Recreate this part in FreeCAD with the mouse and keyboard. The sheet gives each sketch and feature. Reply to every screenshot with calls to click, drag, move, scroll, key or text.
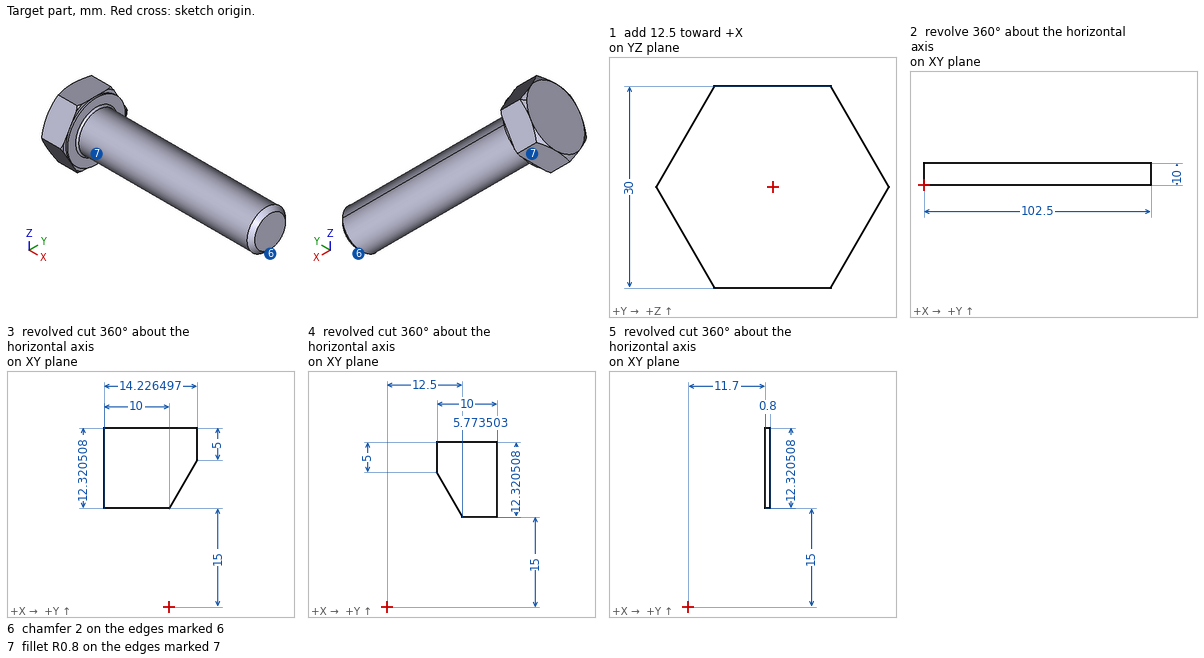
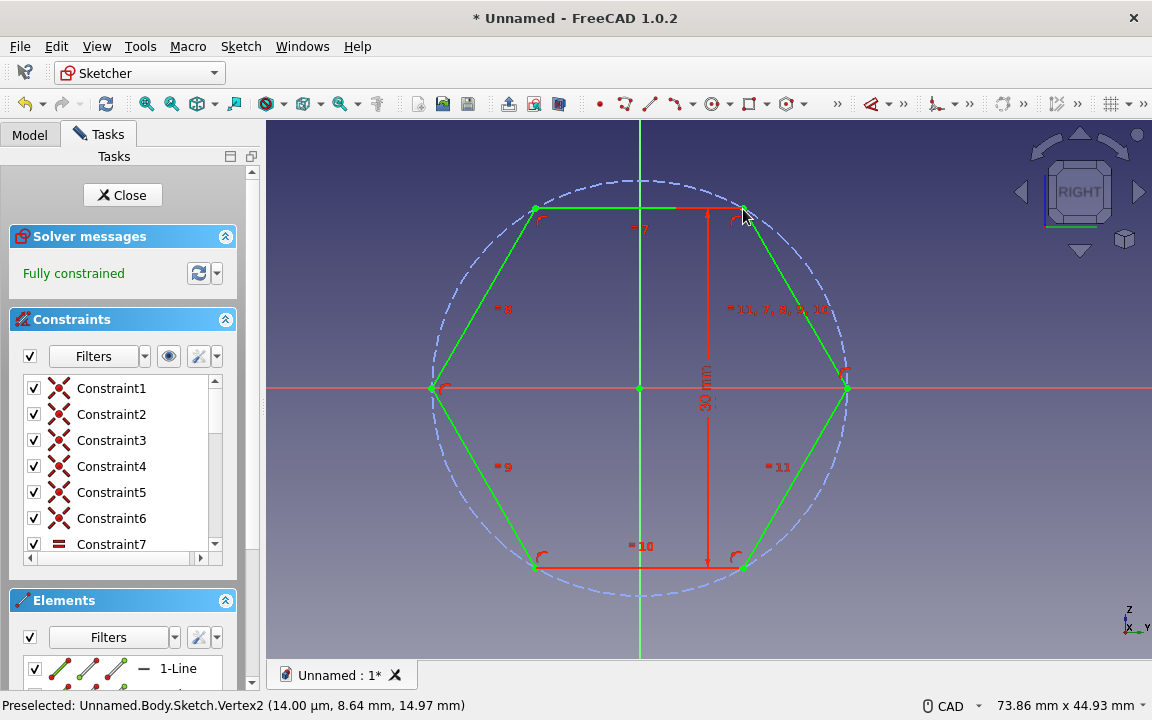
click(123, 195)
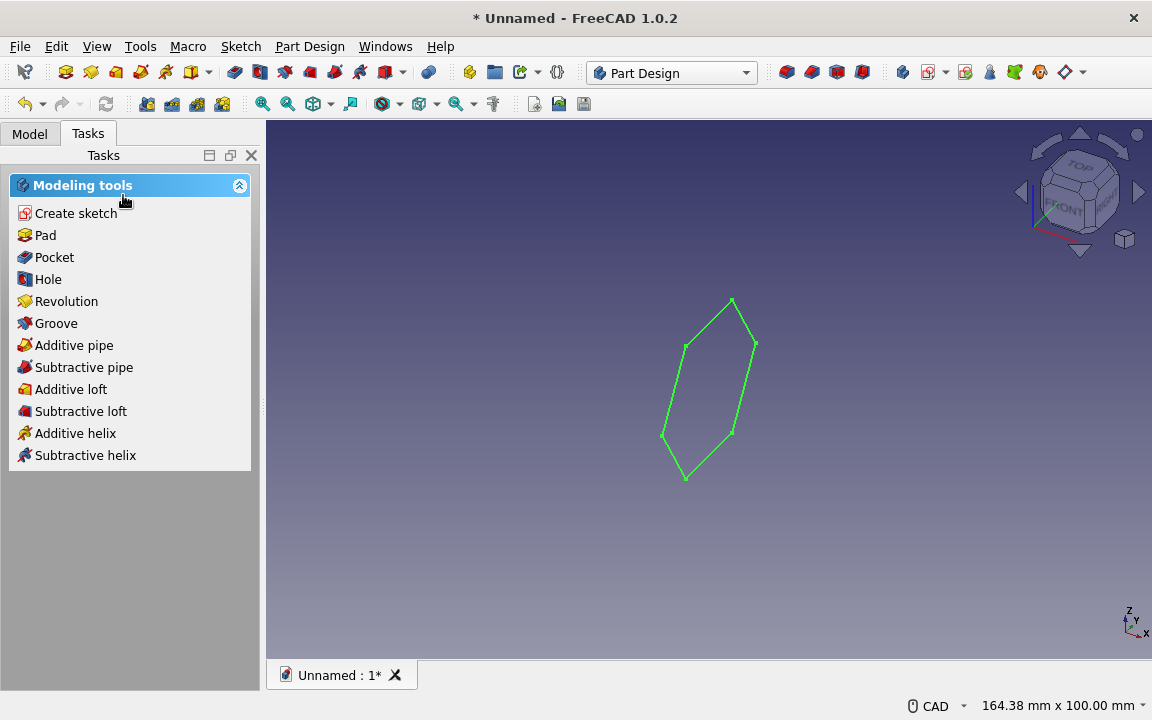
click(66, 72)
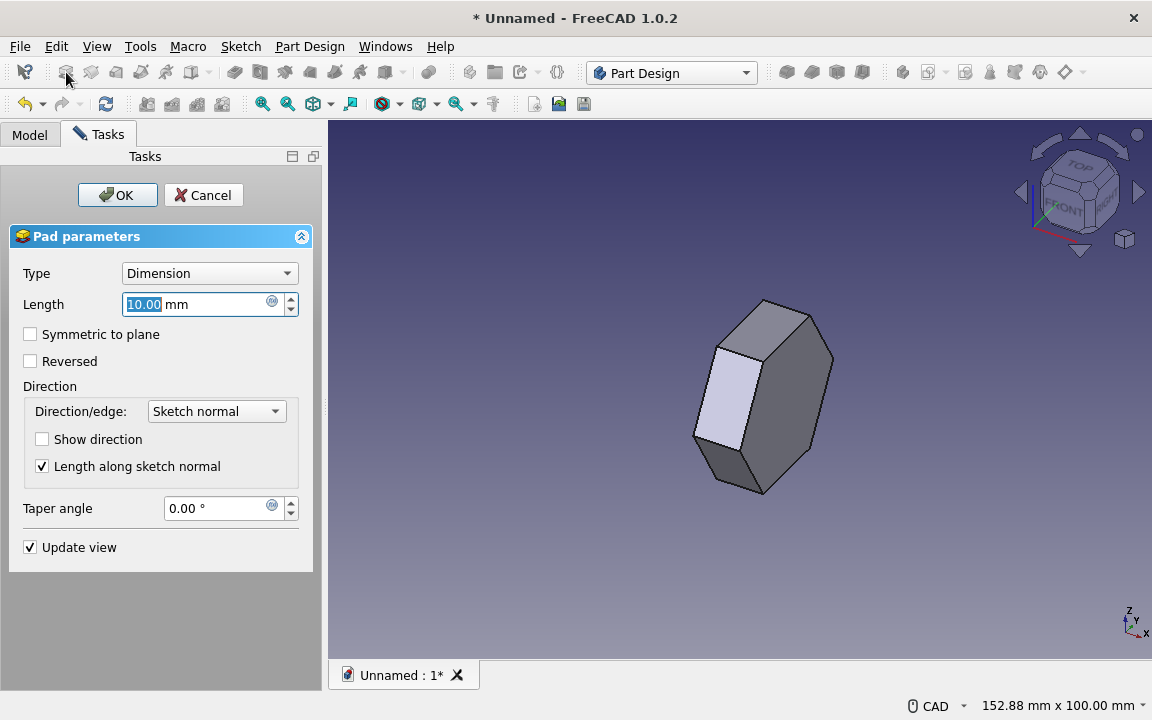
text(12.5)
key(Tab)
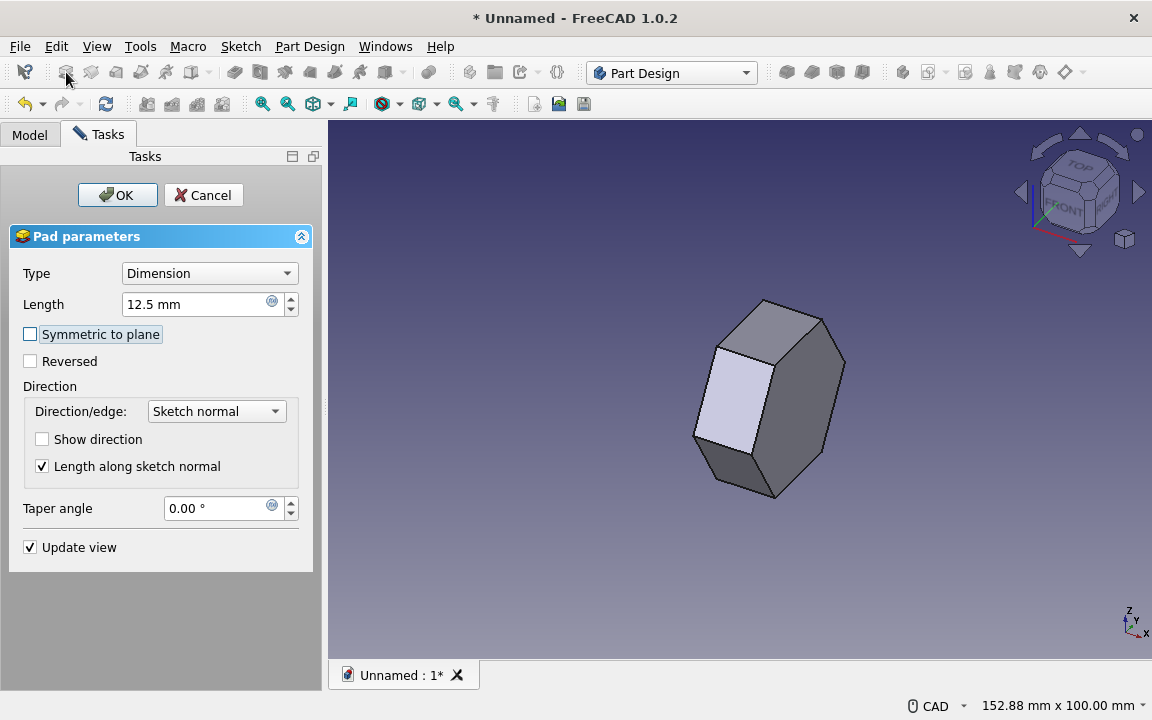
click(118, 195)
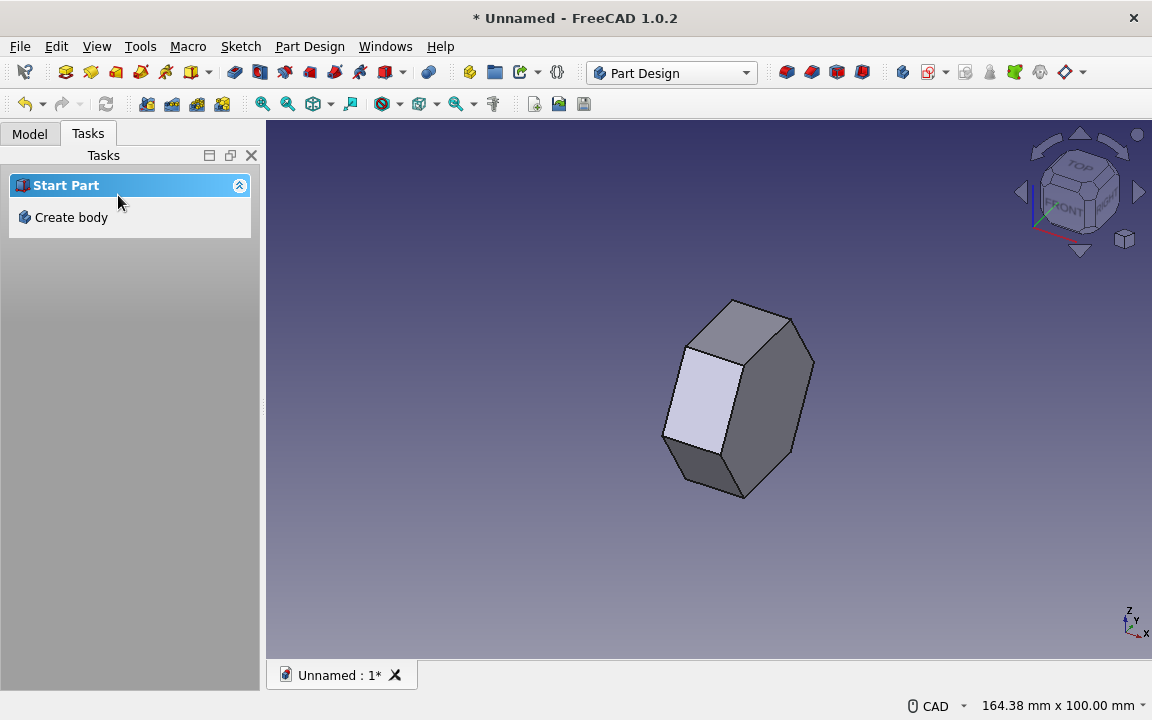
click(928, 72)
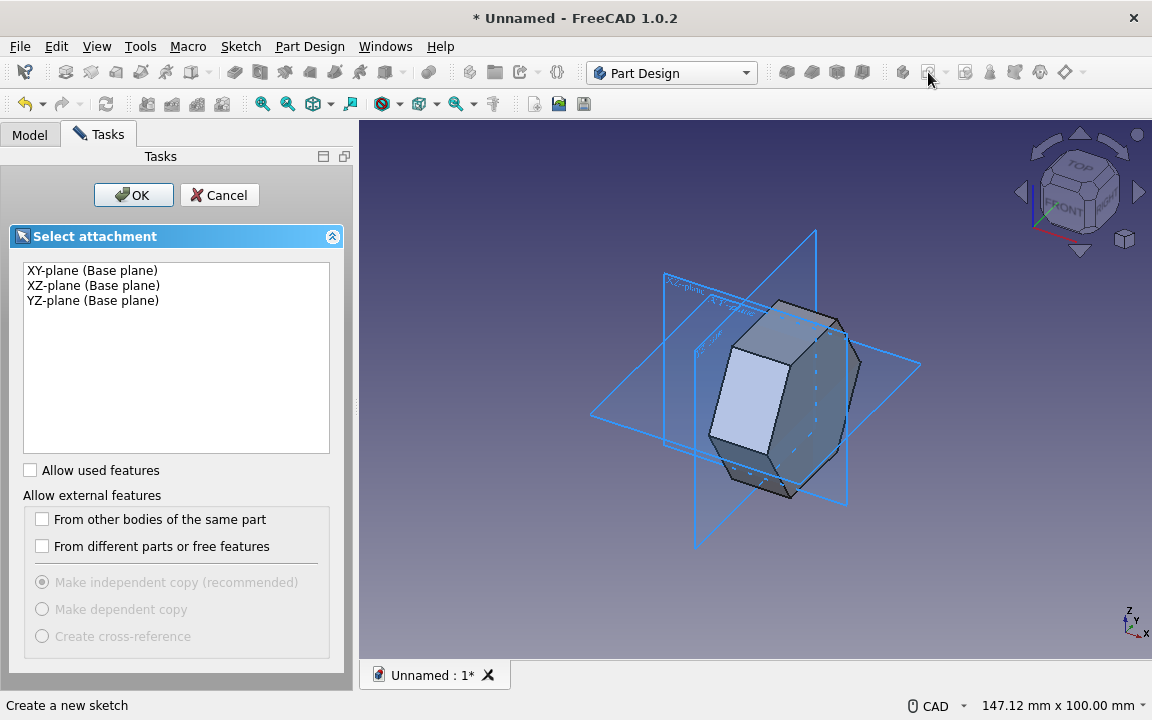
click(84, 270)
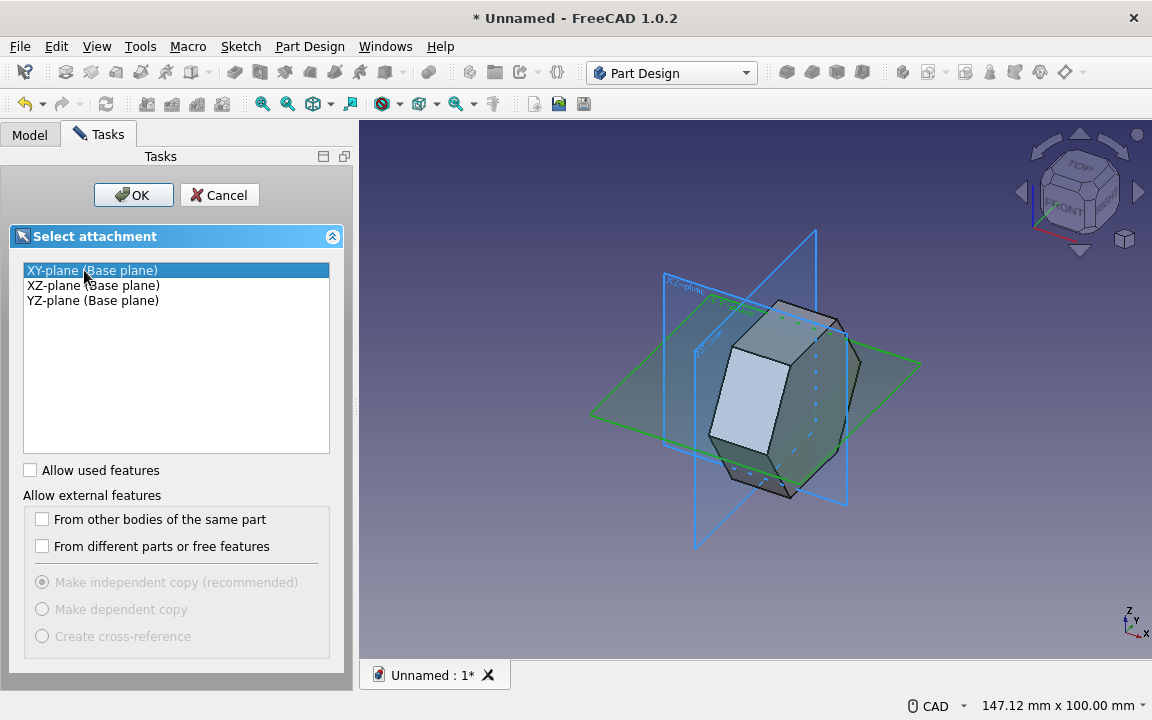
click(134, 195)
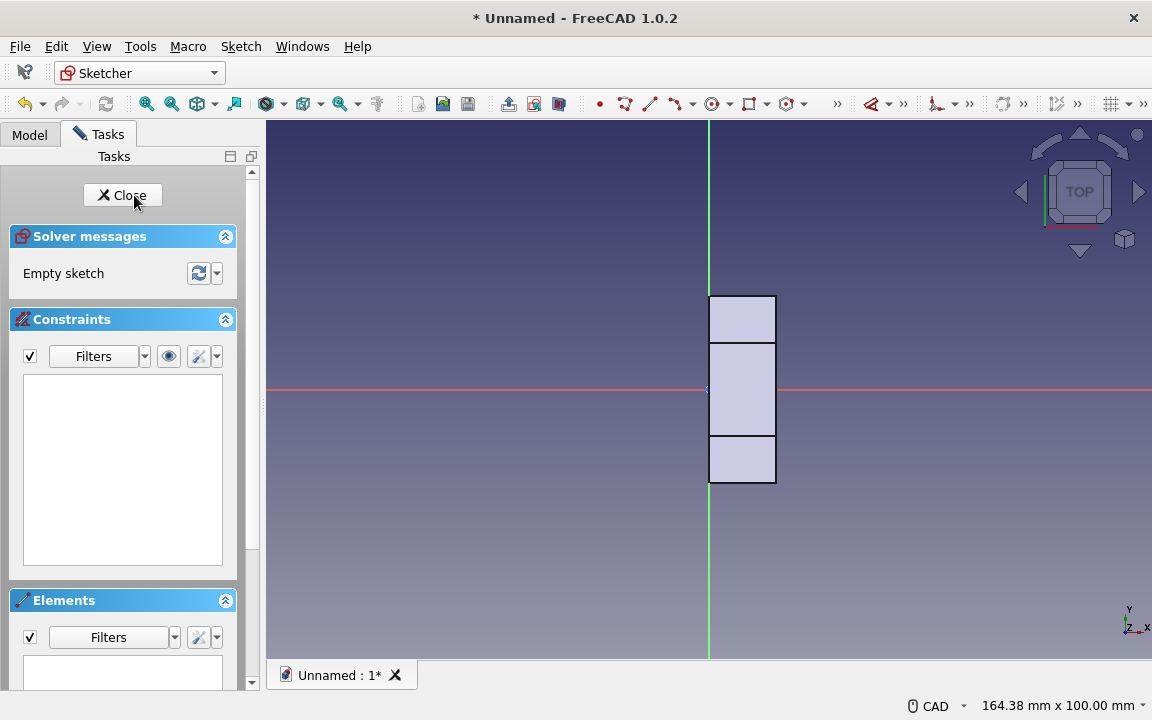
click(559, 104)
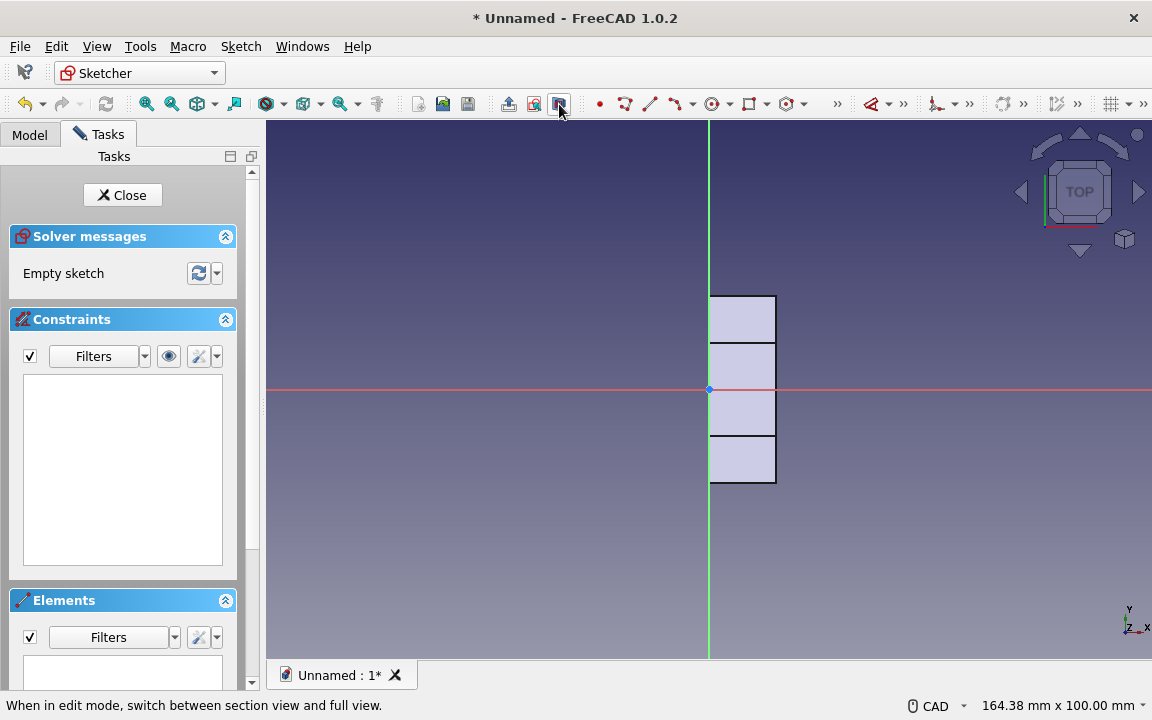
scroll(294, 444, down, 2)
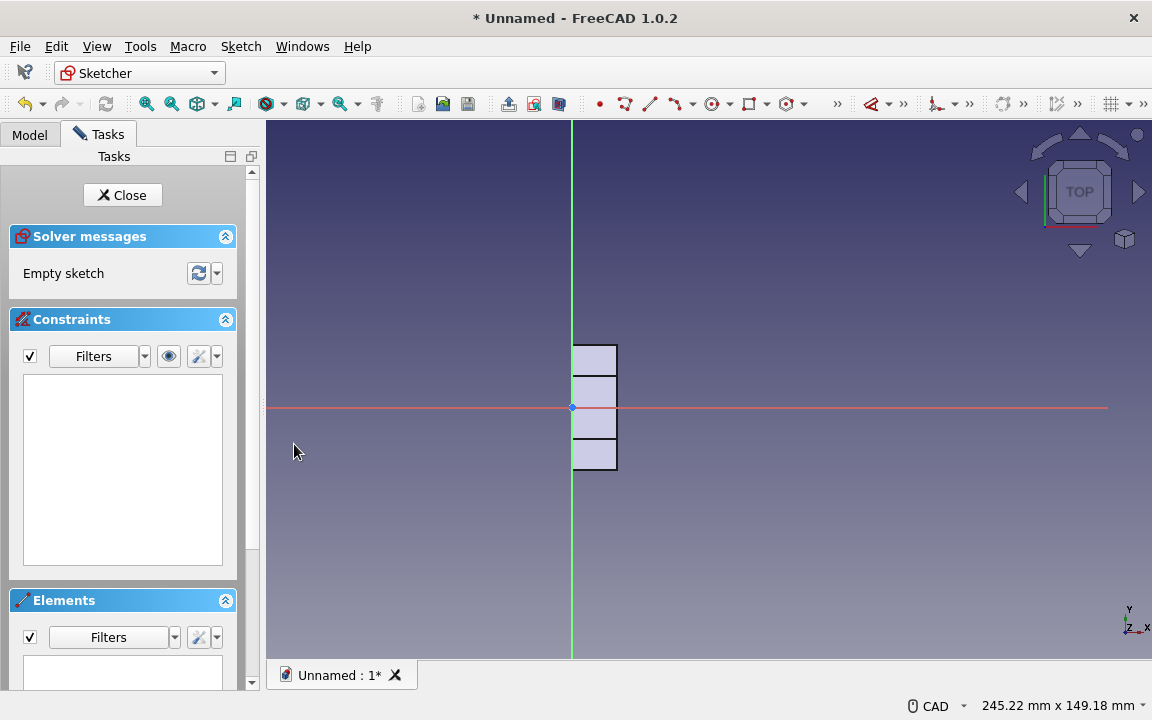
click(748, 104)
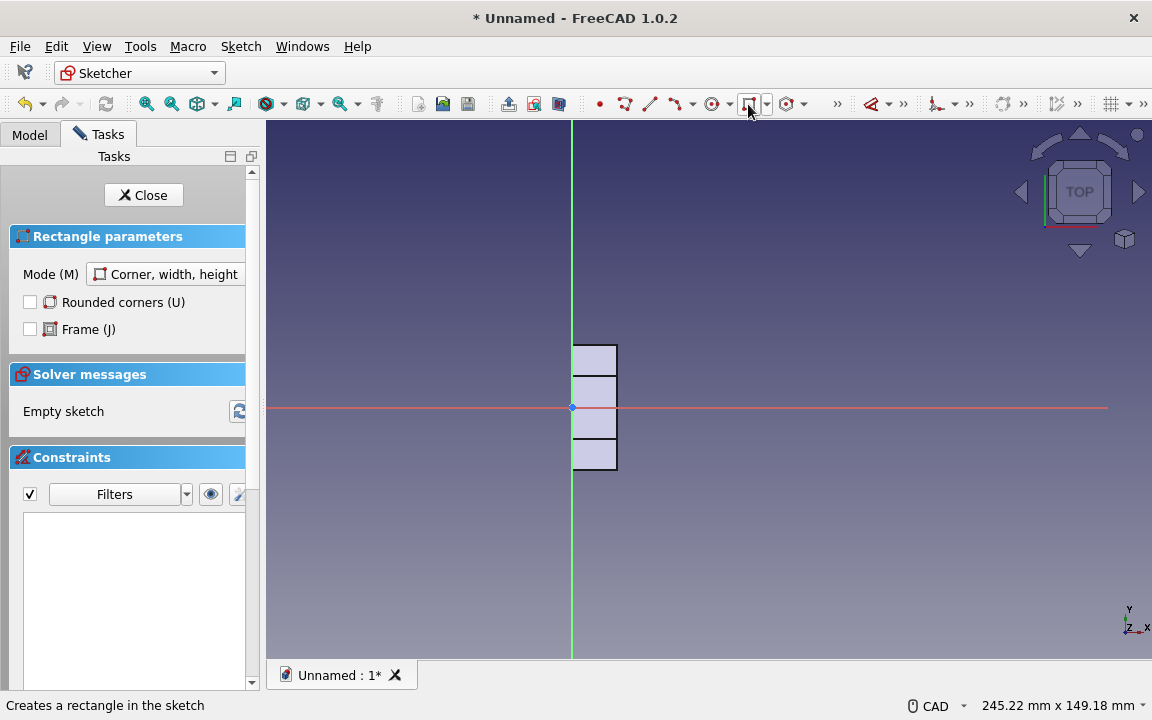
click(572, 408)
move(943, 372)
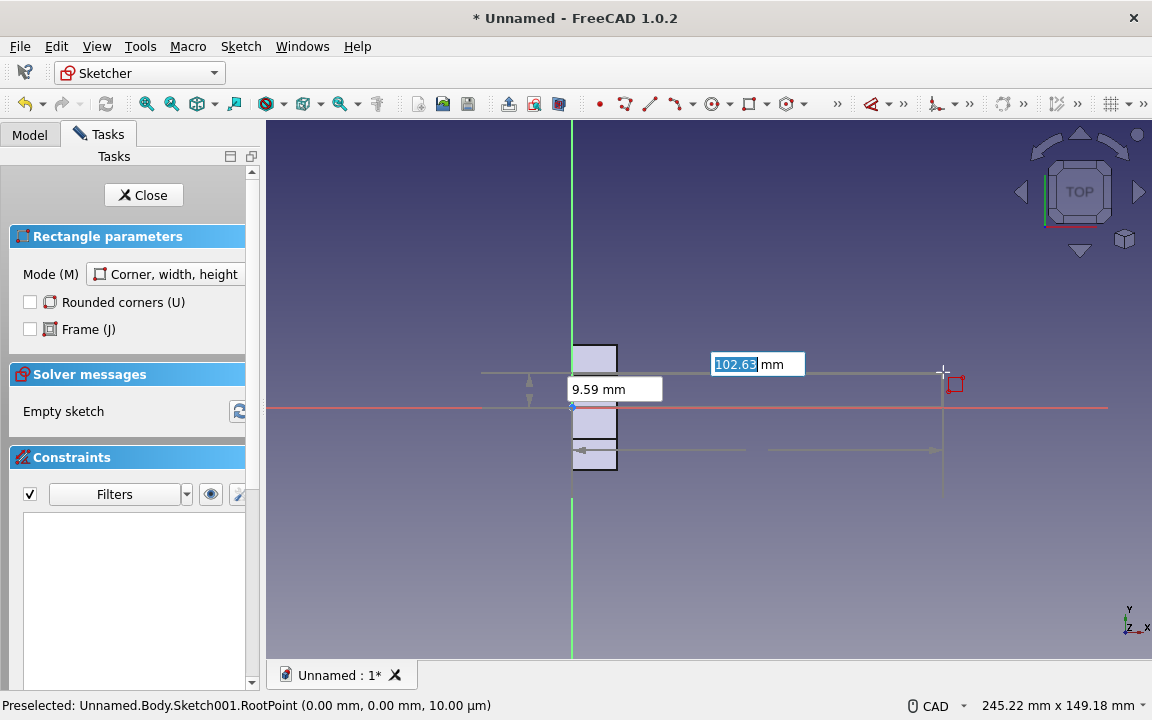
text(102.5)
key(Tab)
text(10)
key(Return)
key(Escape)